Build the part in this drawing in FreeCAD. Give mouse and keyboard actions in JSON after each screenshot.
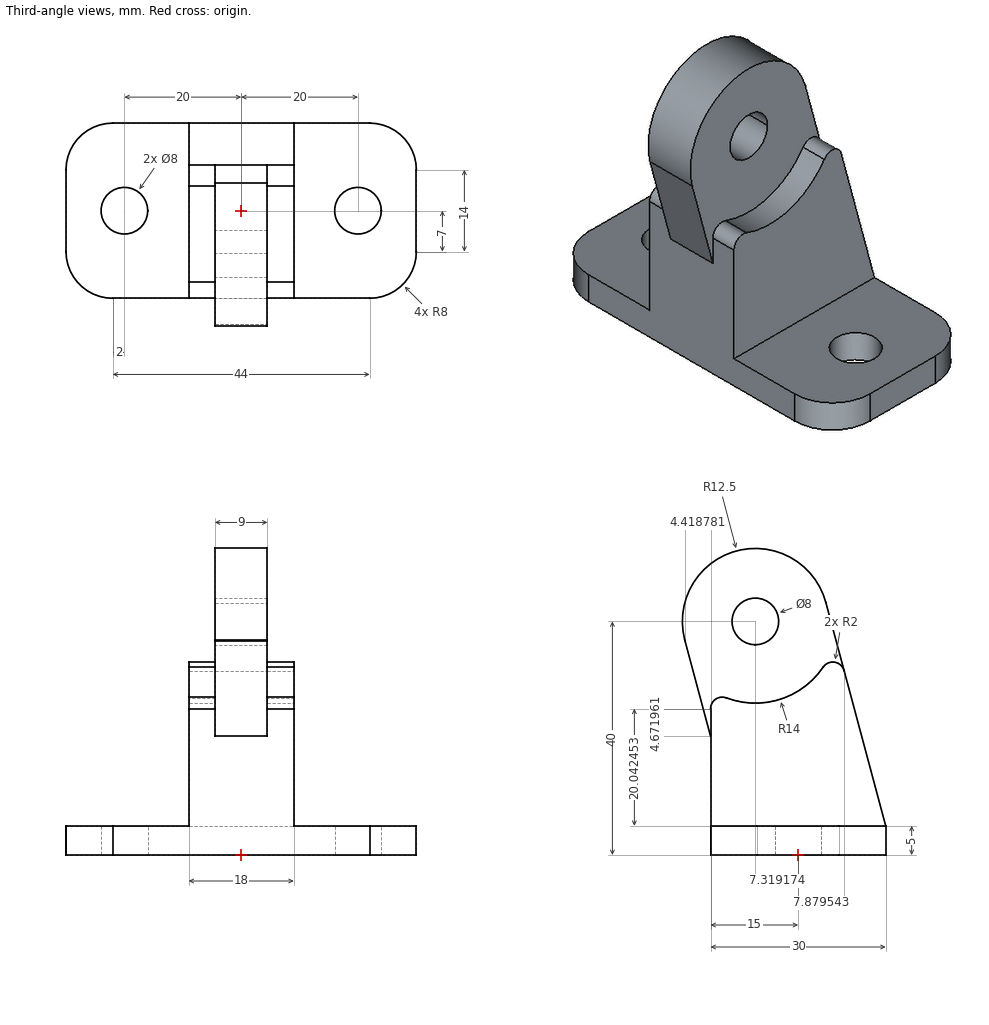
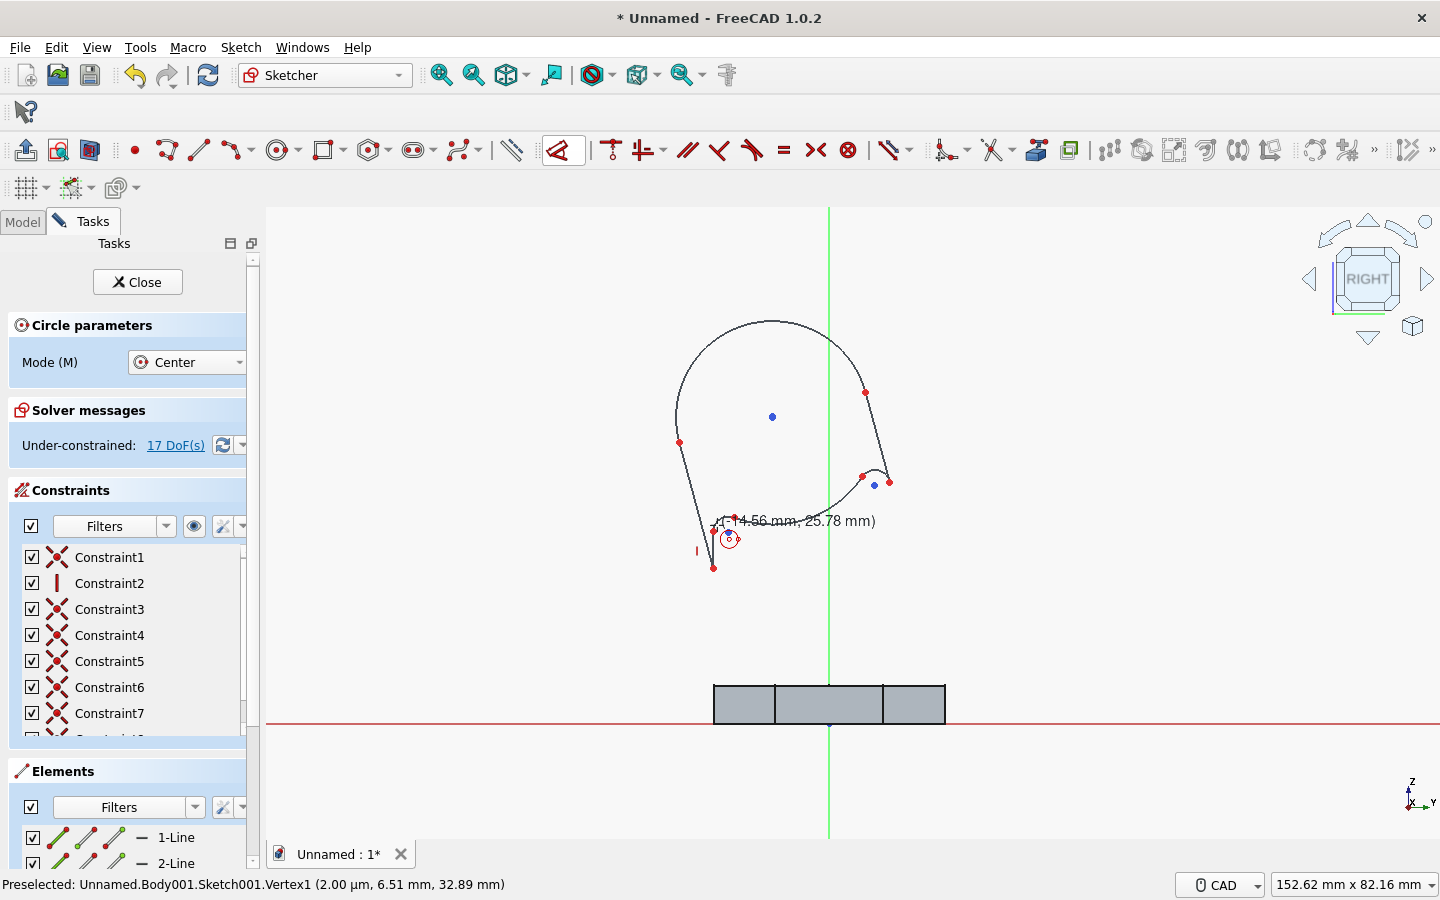
{"action": "left_click", "coordinate": [773, 416]}
{"action": "left_click", "coordinate": [795, 395]}
{"action": "key", "text": "Escape"}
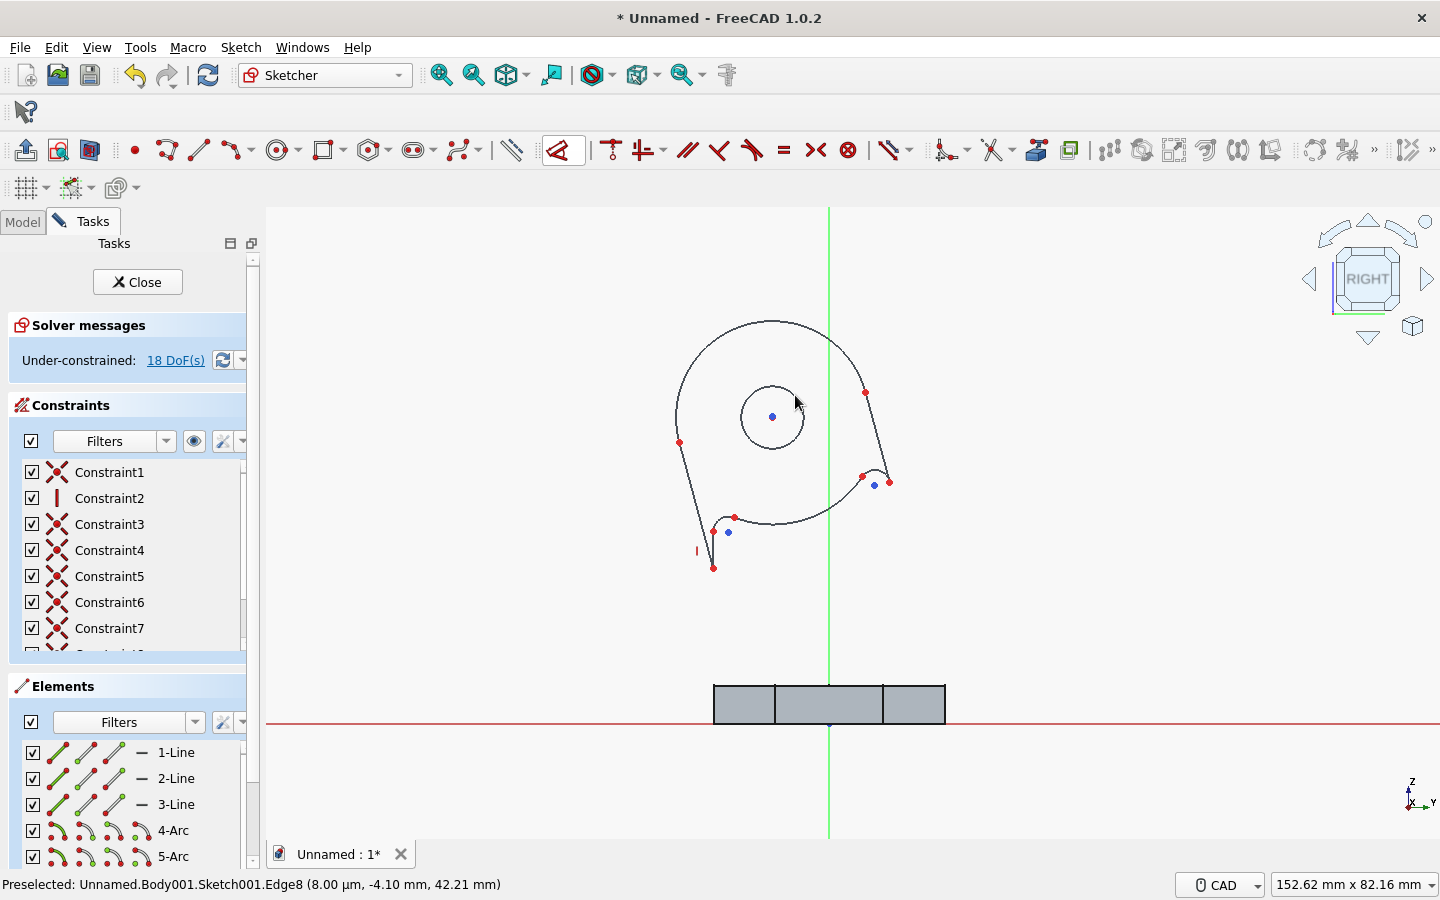
{"action": "left_click", "coordinate": [883, 455]}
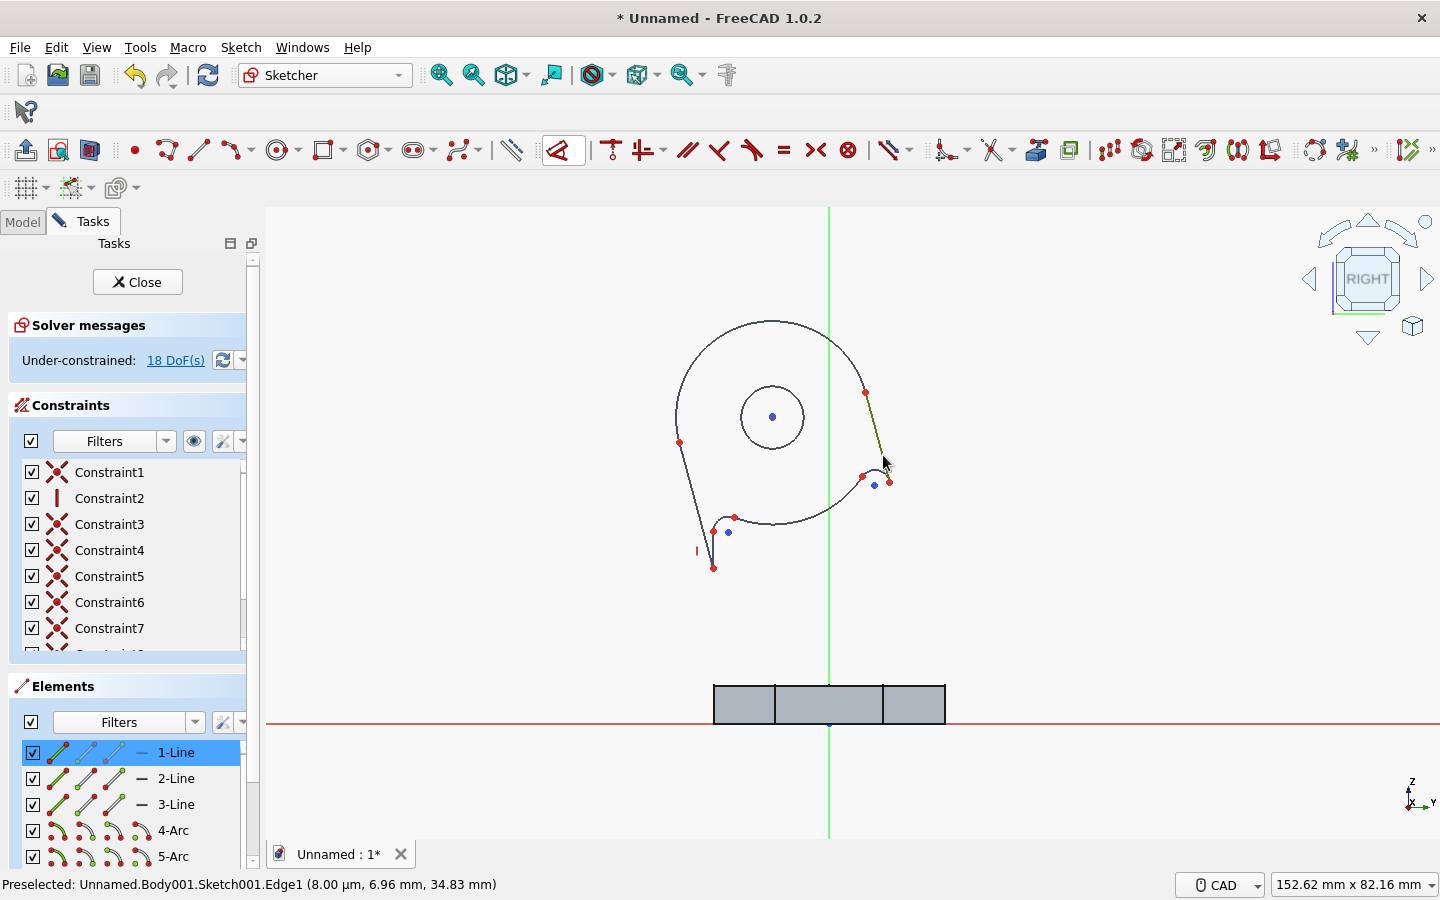
{"action": "left_click", "coordinate": [807, 327]}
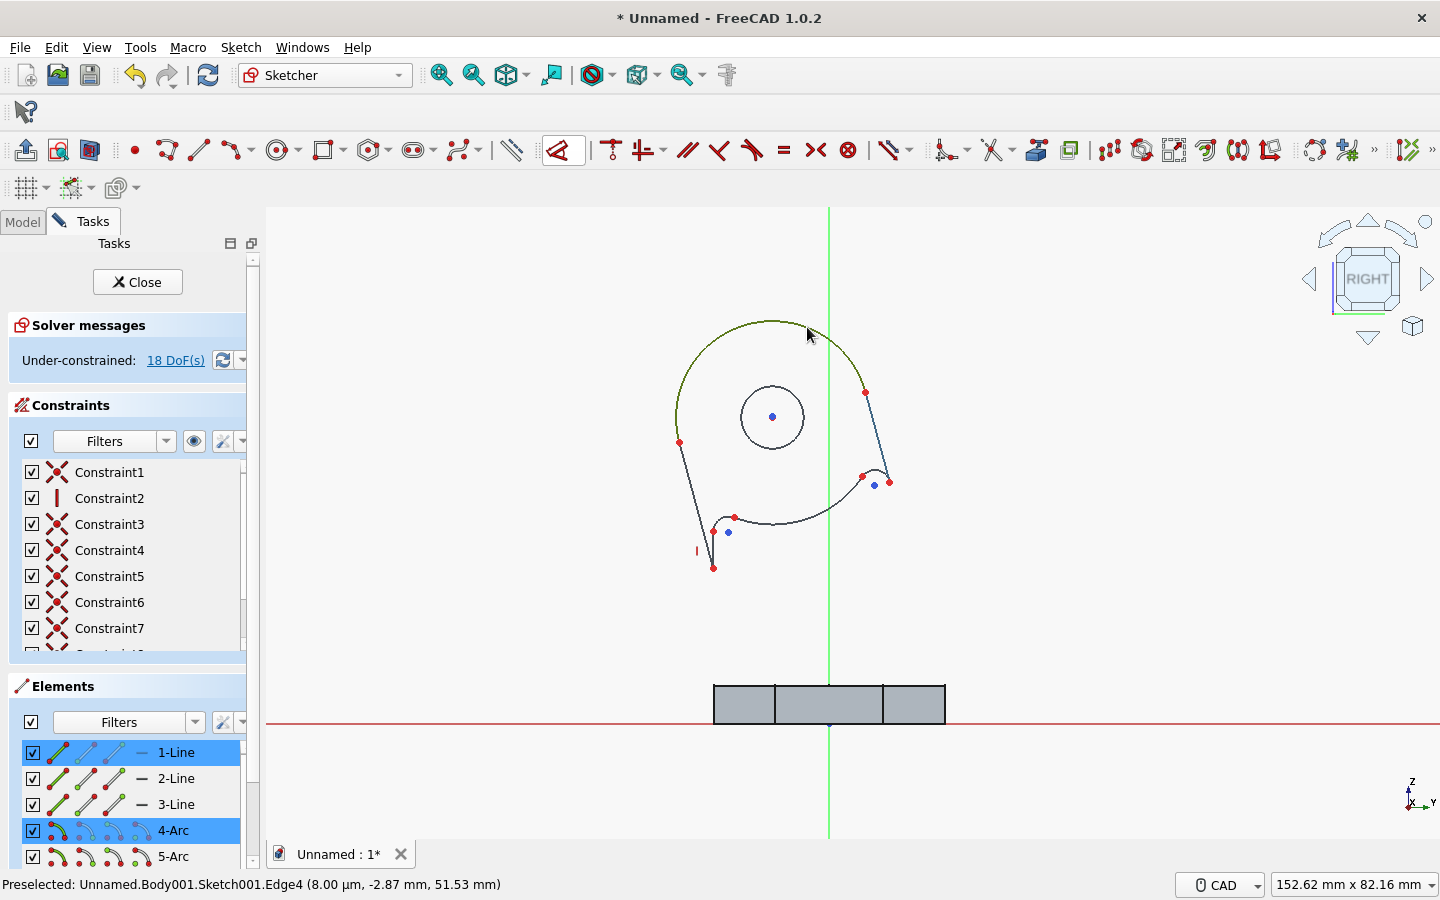
{"action": "key", "text": "t"}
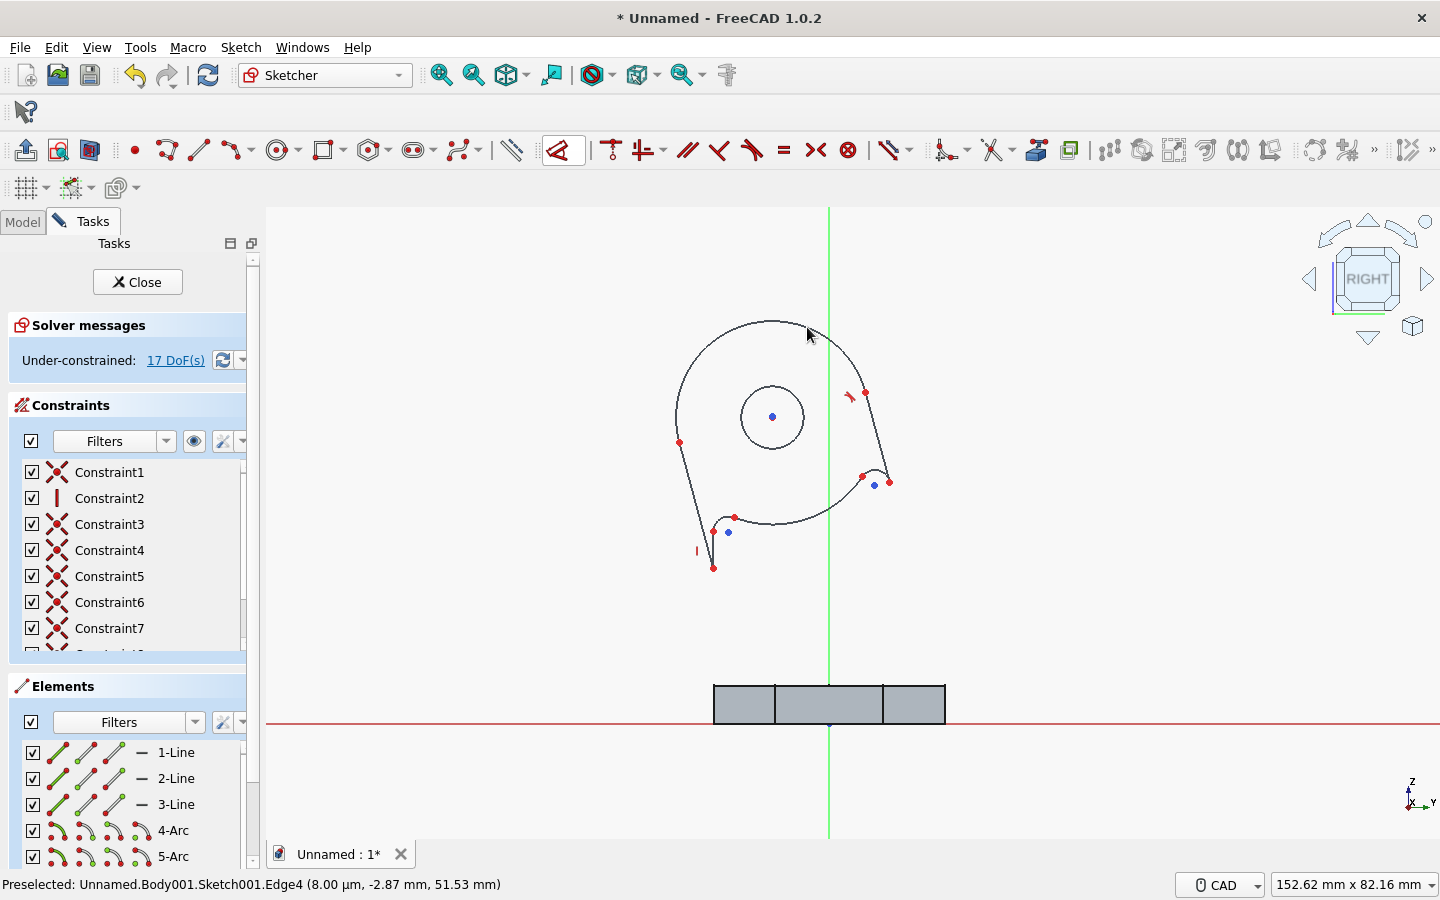
{"action": "left_click", "coordinate": [883, 455]}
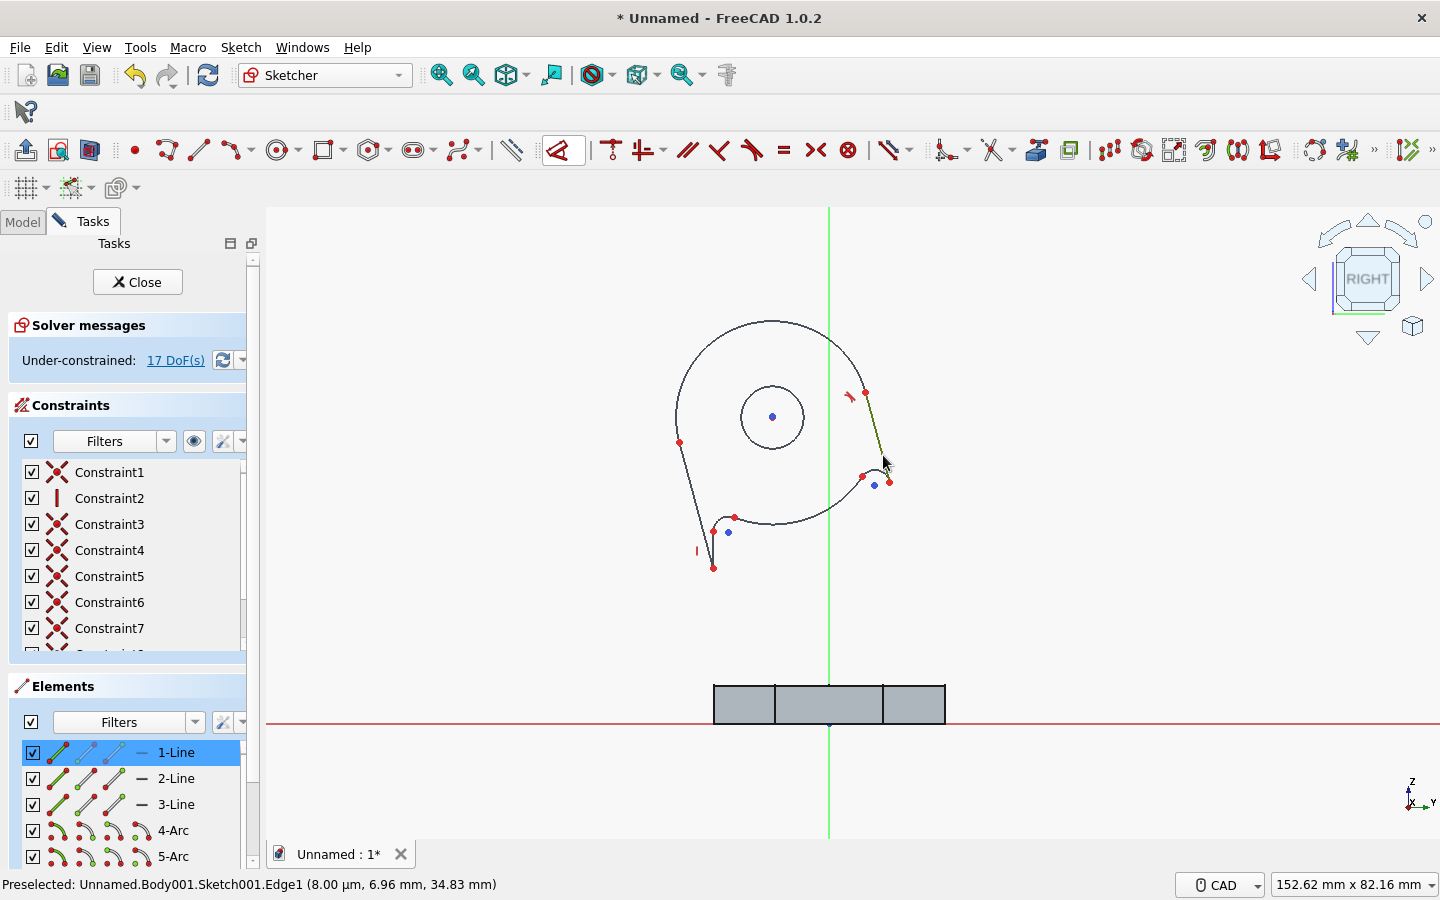
{"action": "scroll", "coordinate": [871, 471], "scroll_direction": "up", "scroll_amount": 2}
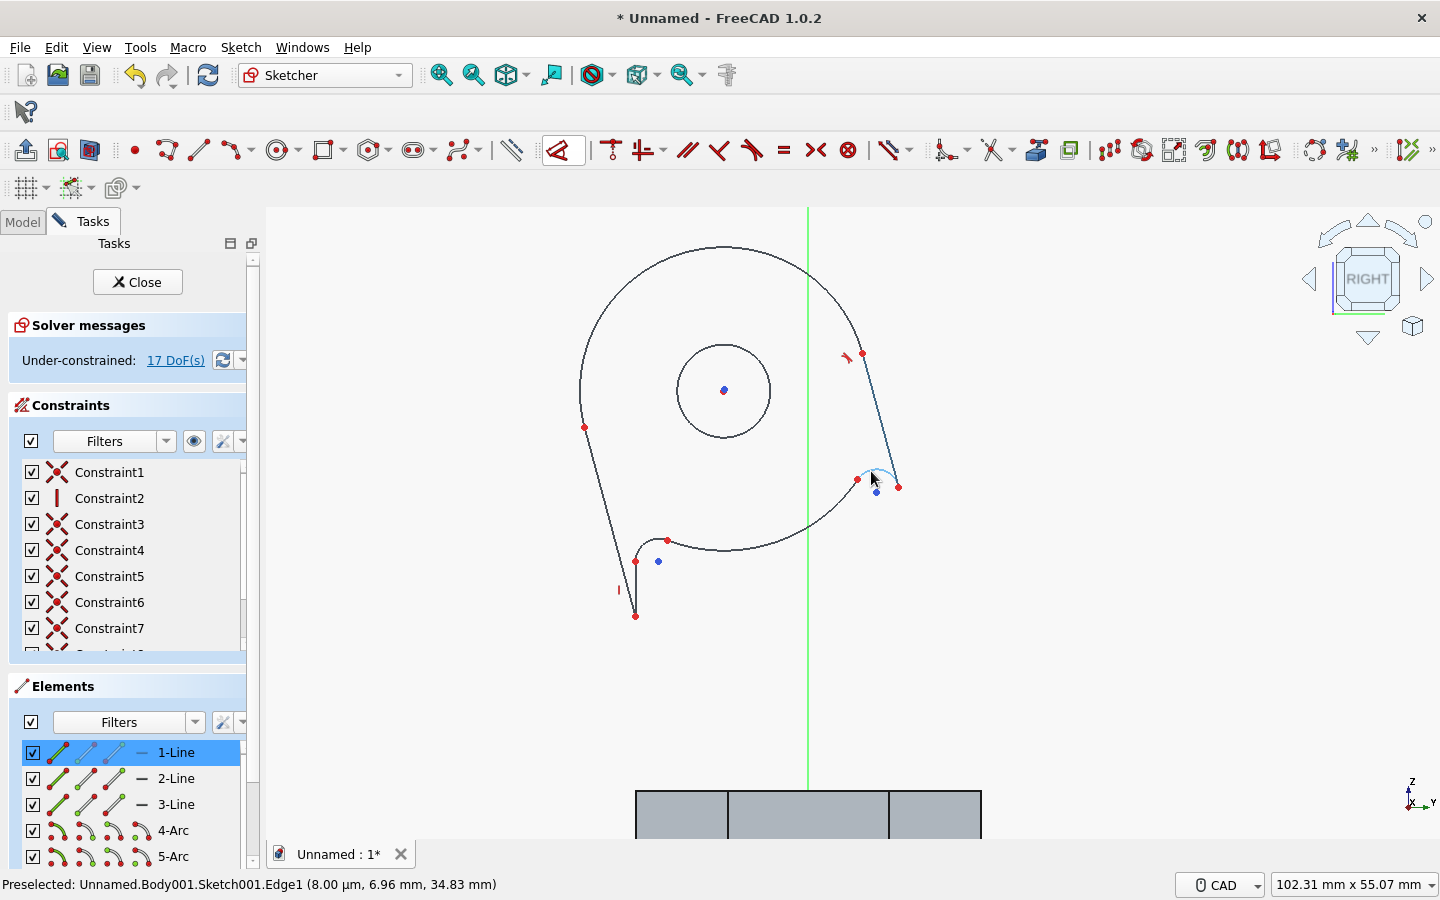
{"action": "left_click", "coordinate": [870, 470]}